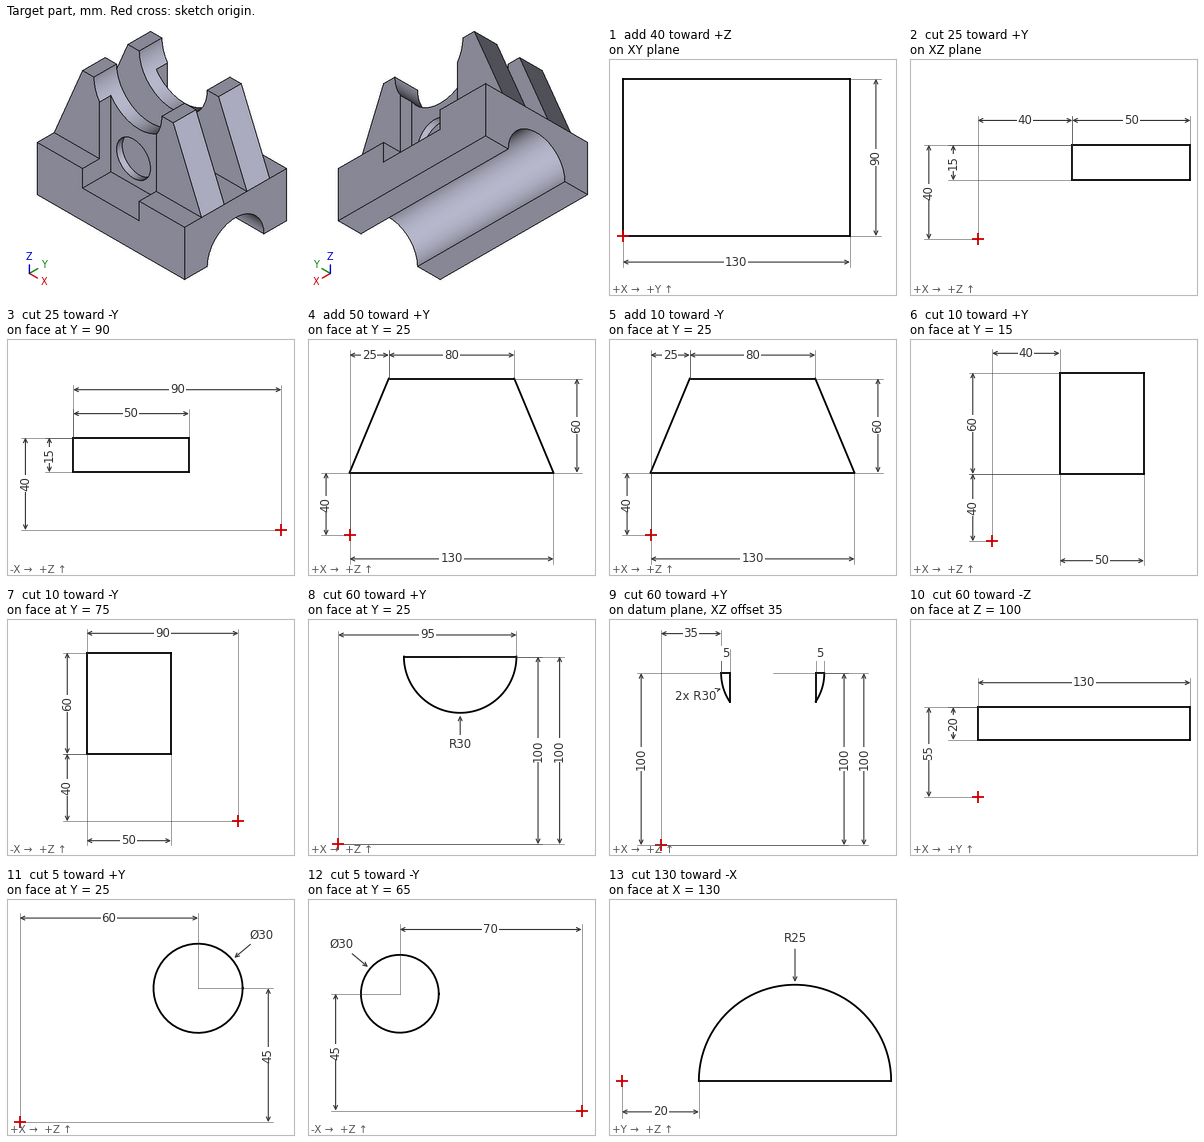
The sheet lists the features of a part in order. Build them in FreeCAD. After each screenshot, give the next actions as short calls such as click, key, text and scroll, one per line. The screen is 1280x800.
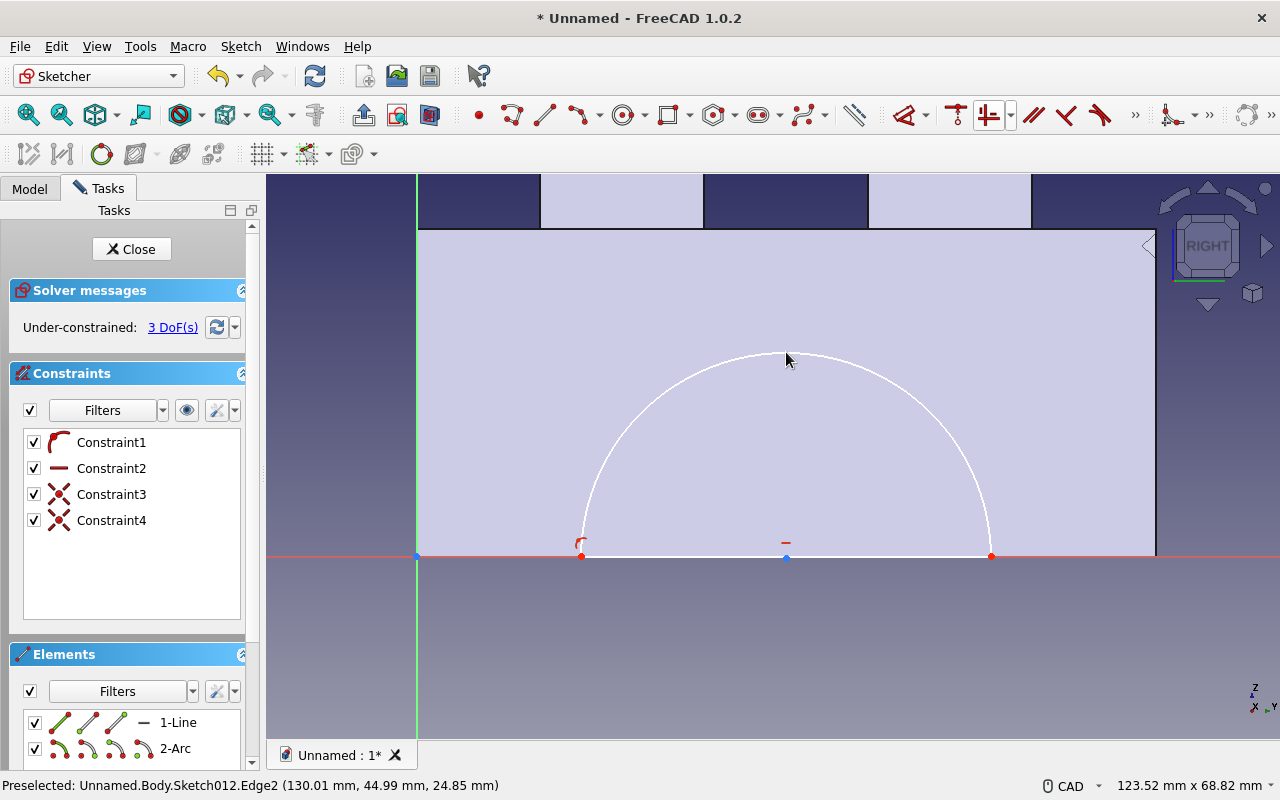
click(786, 558)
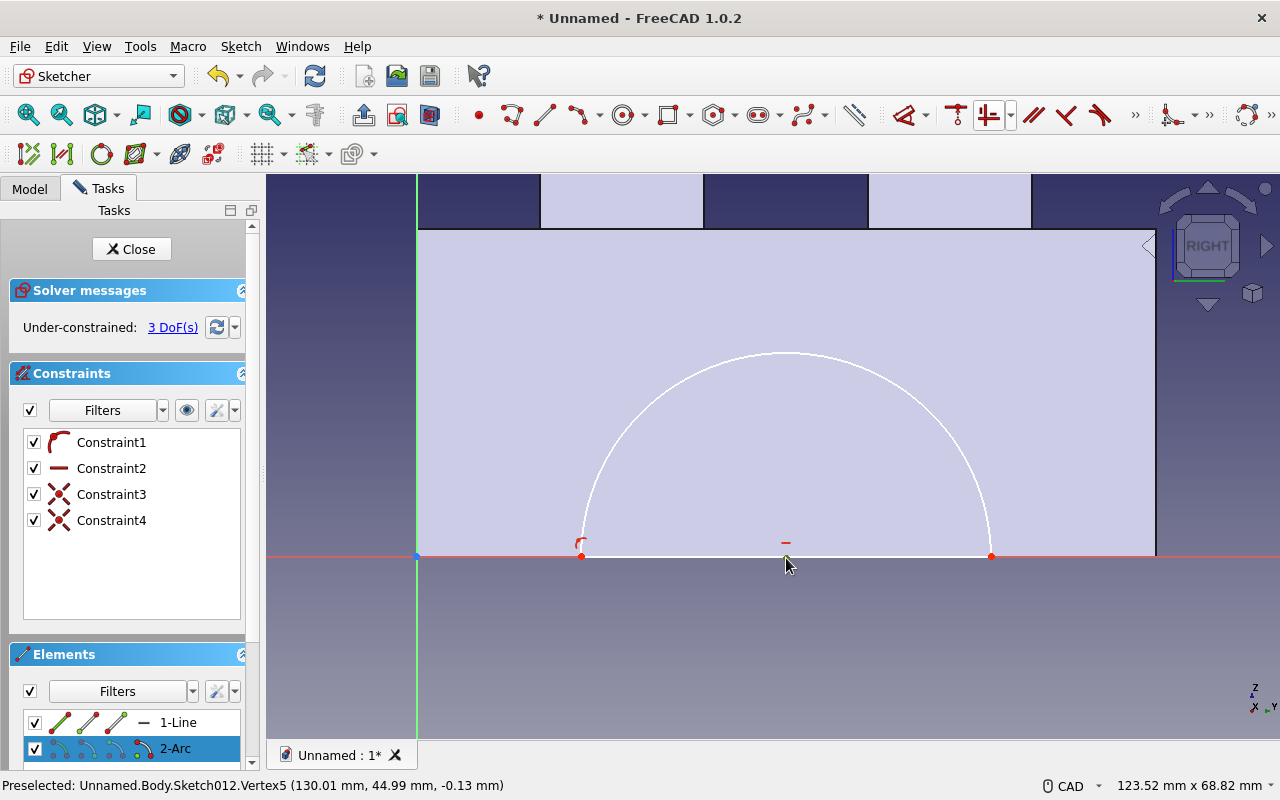
click(353, 557)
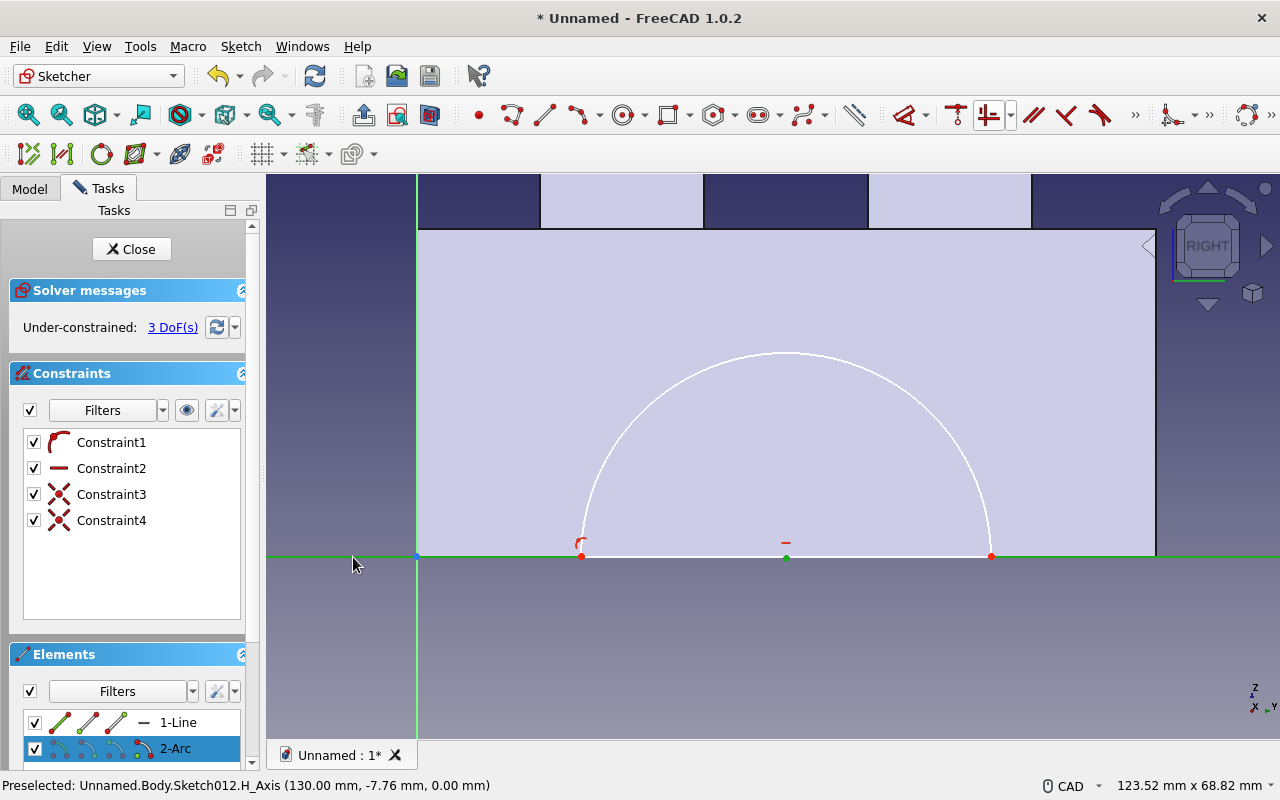
key(c)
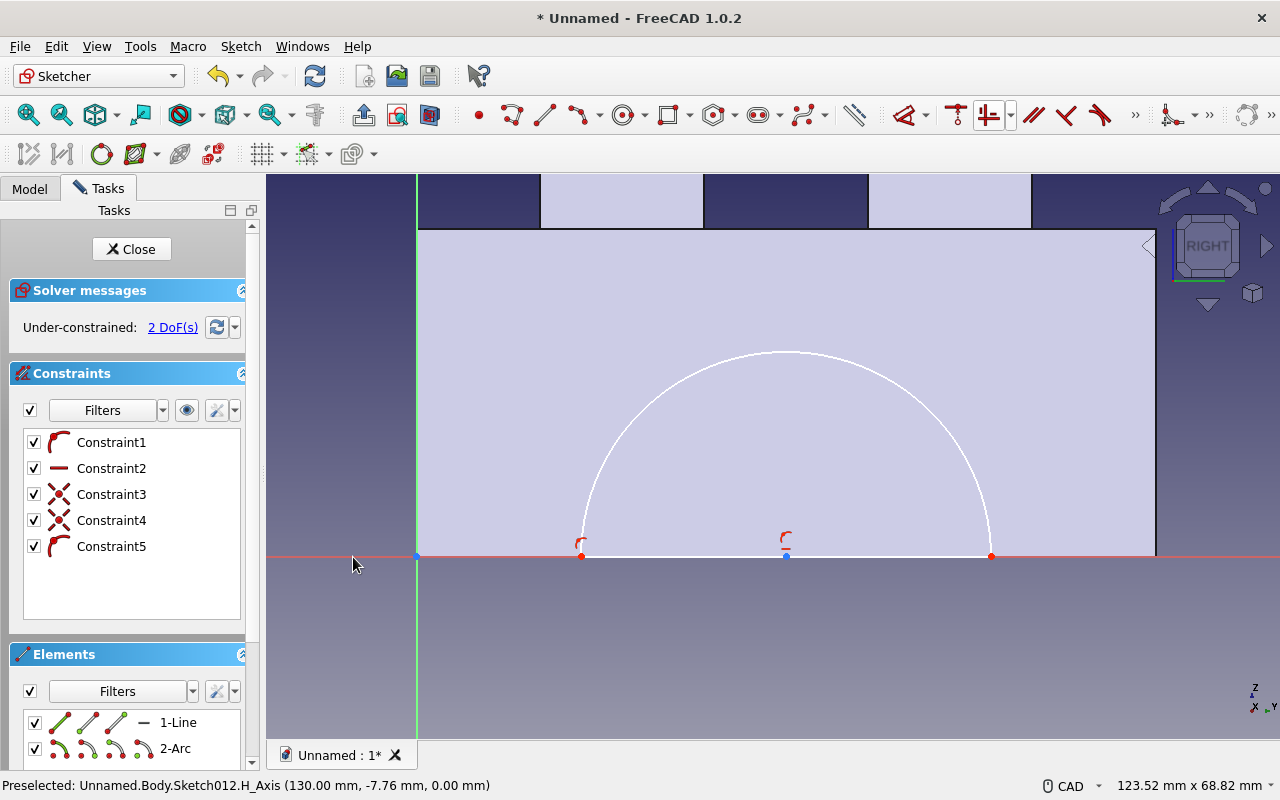
key(d)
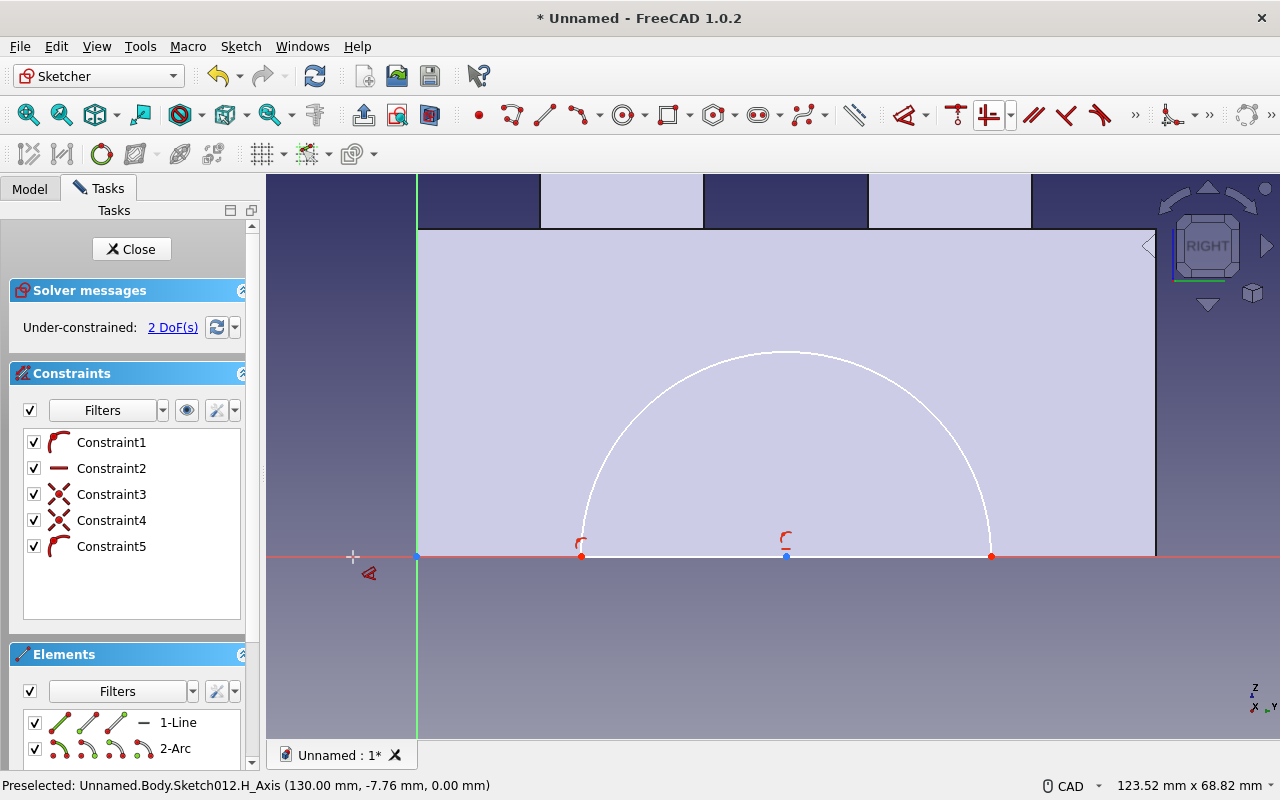
click(906, 391)
click(925, 365)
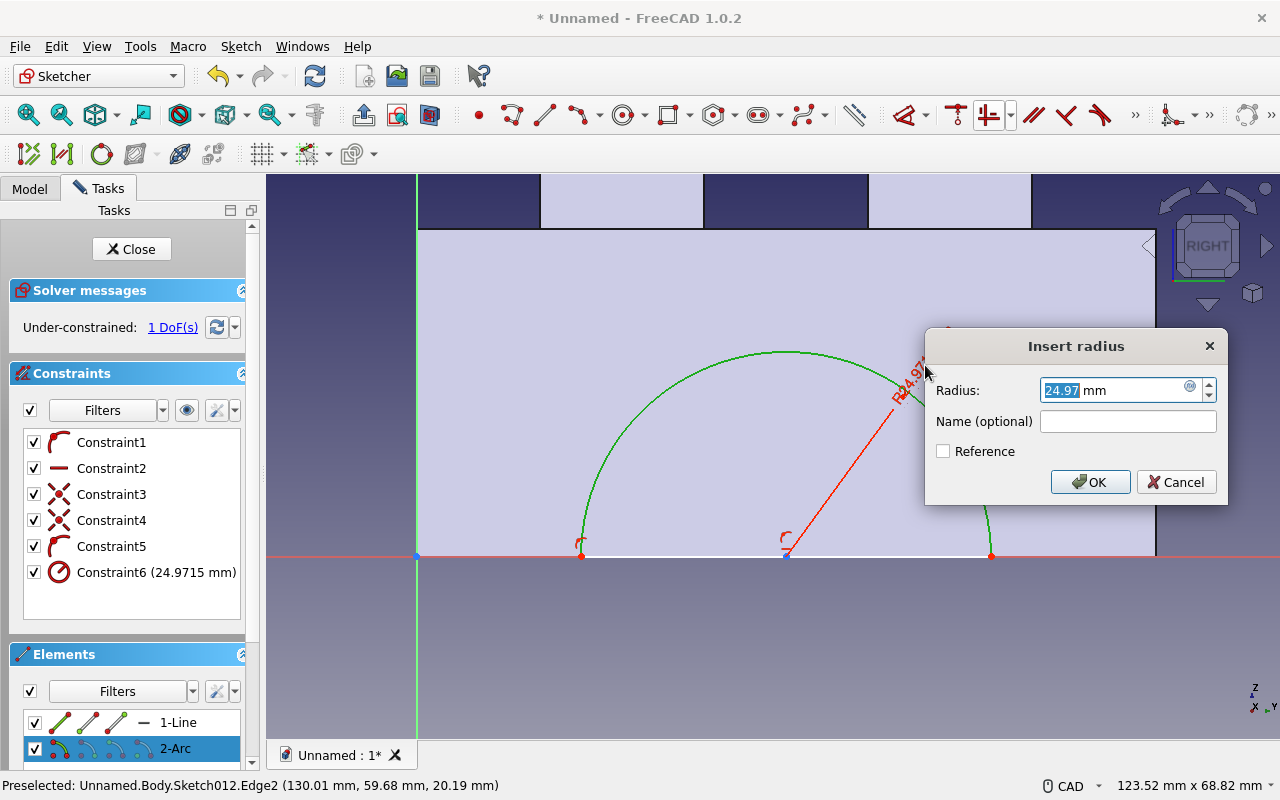
text(25)
key(Return)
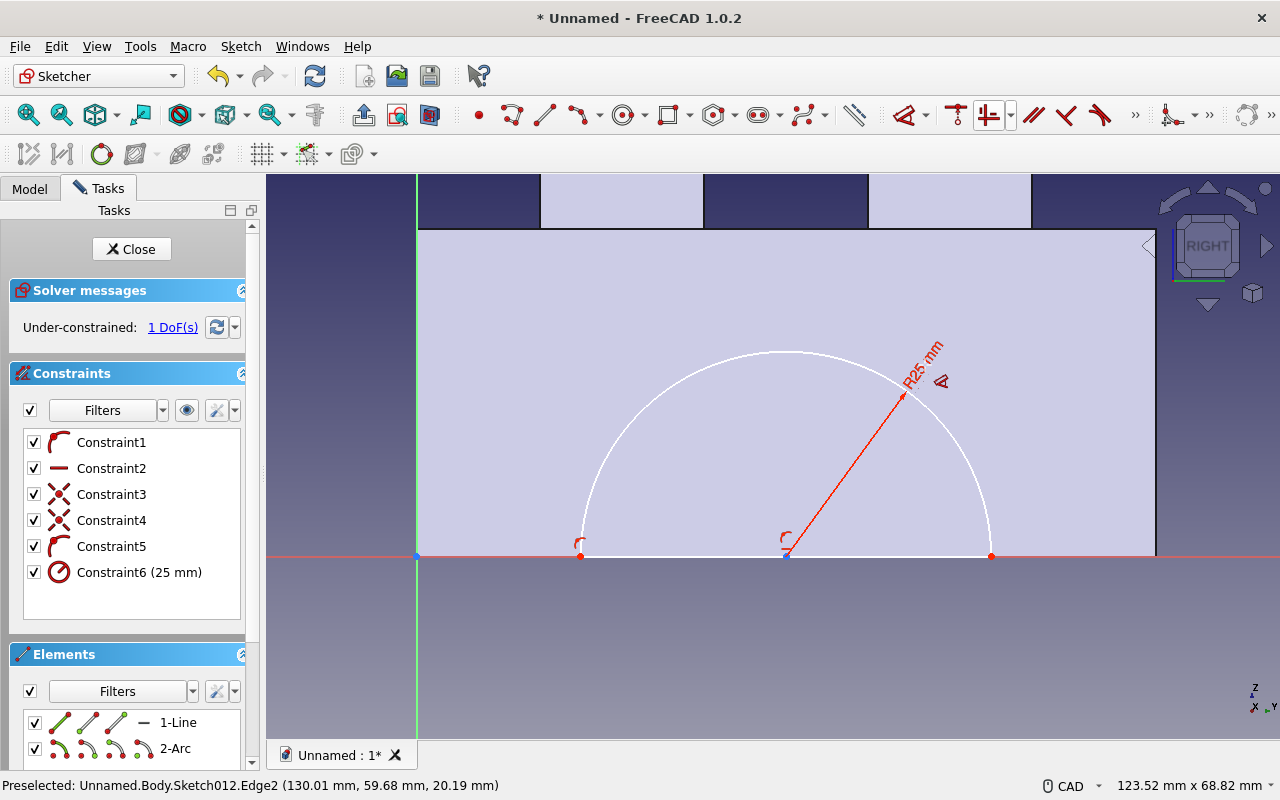
click(581, 557)
click(499, 591)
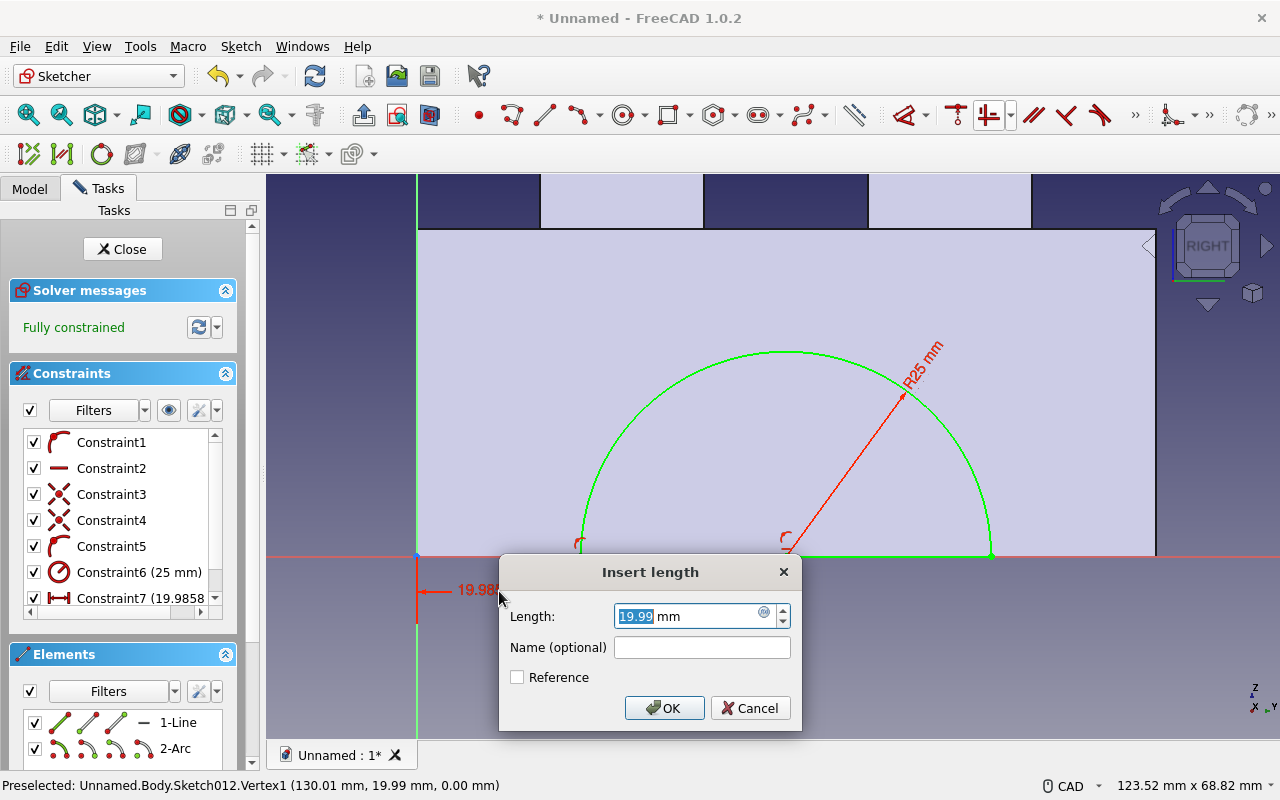
text(20)
key(Return)
key(Escape)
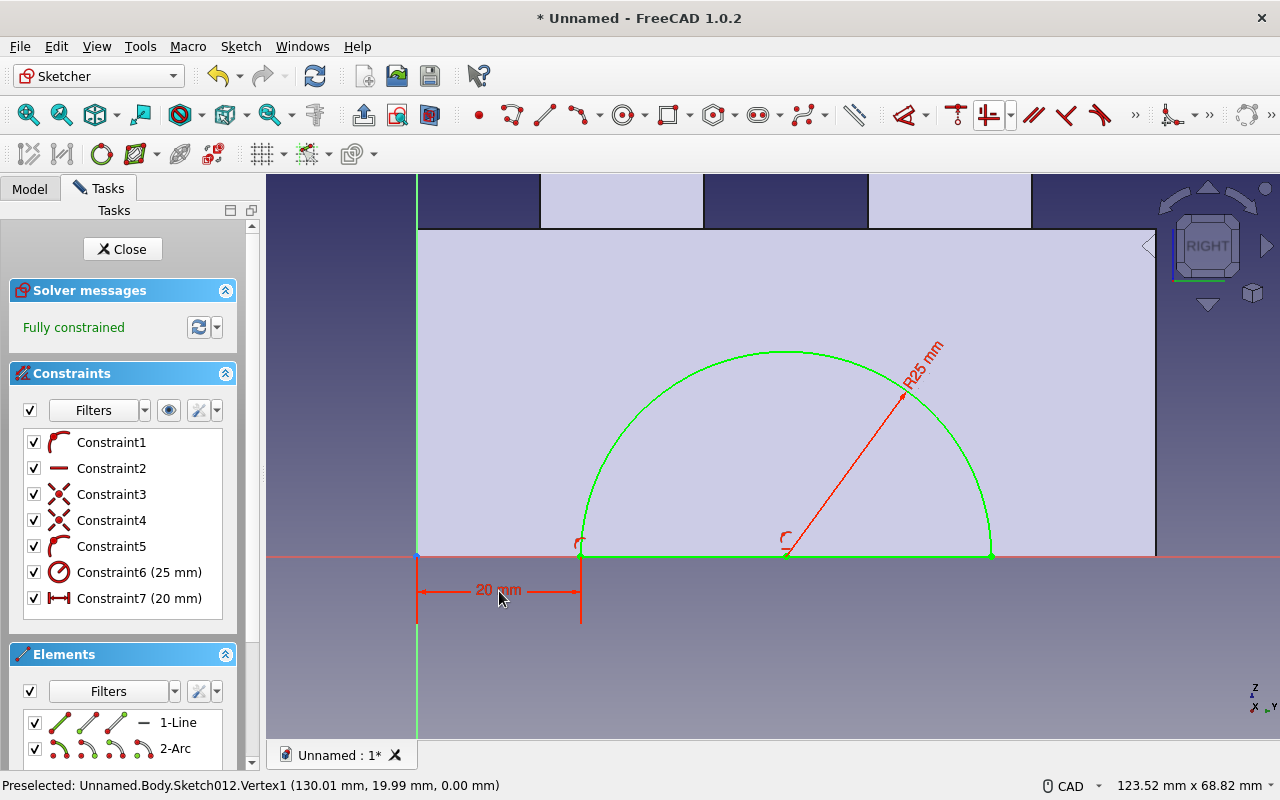
click(123, 249)